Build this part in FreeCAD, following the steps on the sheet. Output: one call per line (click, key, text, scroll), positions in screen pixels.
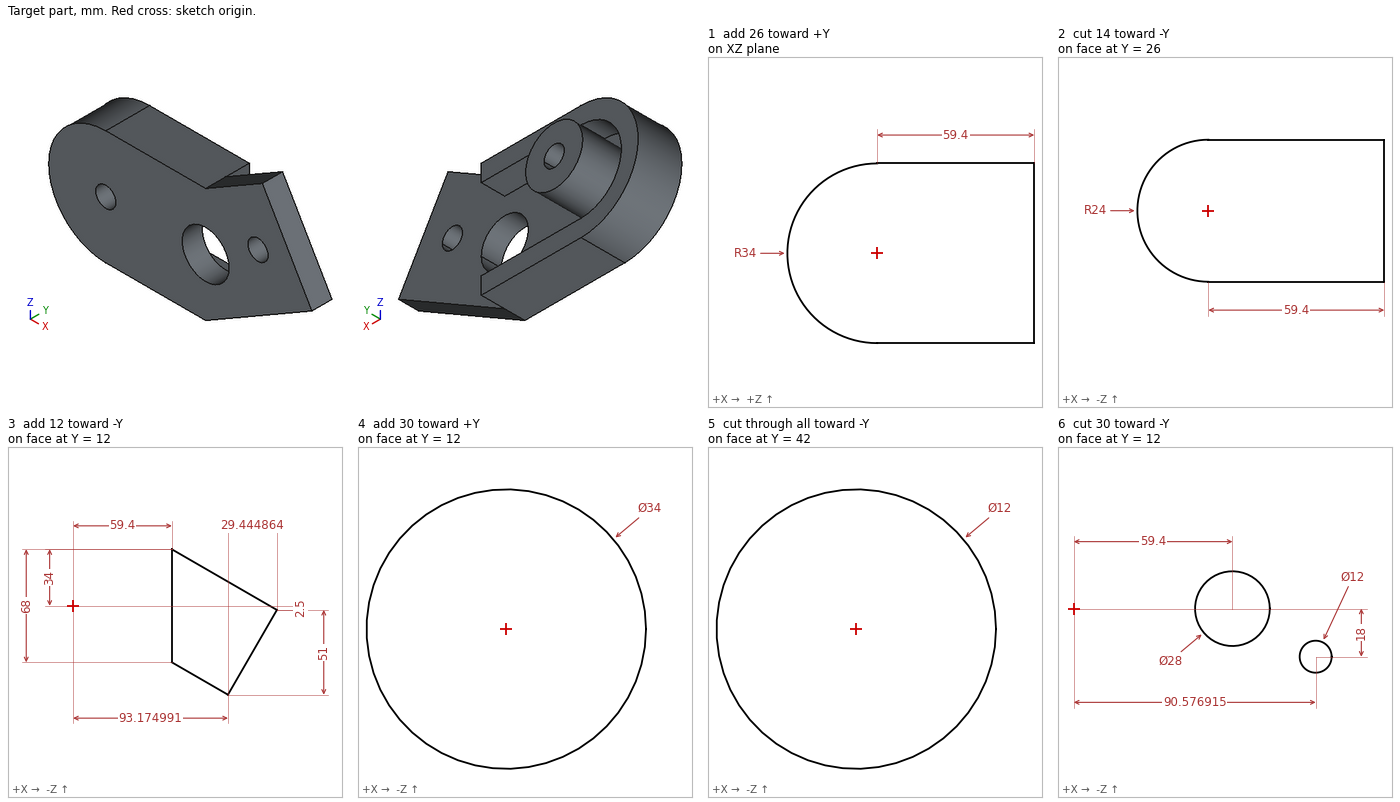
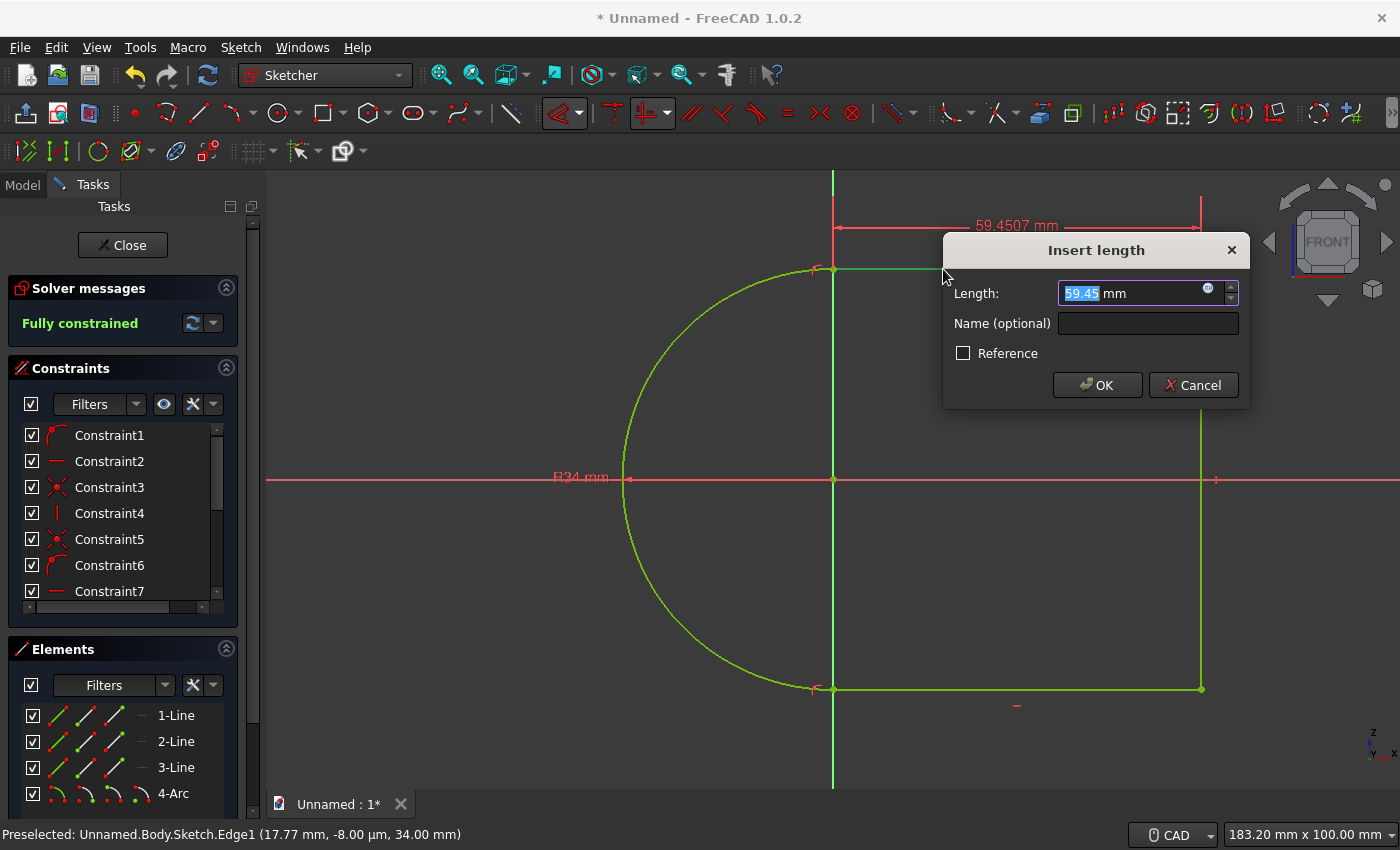
text(59.4)
key(Return)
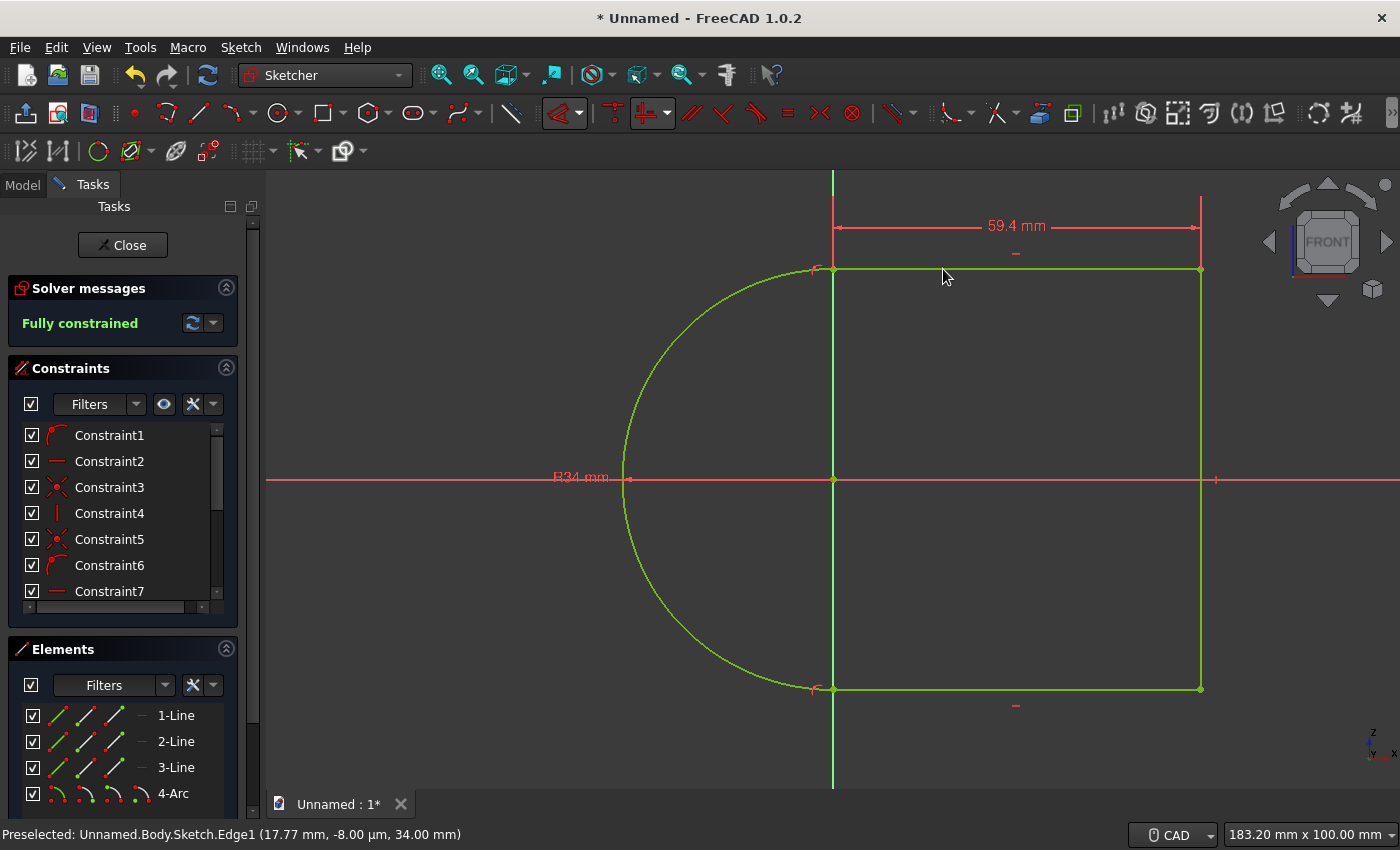
click(123, 245)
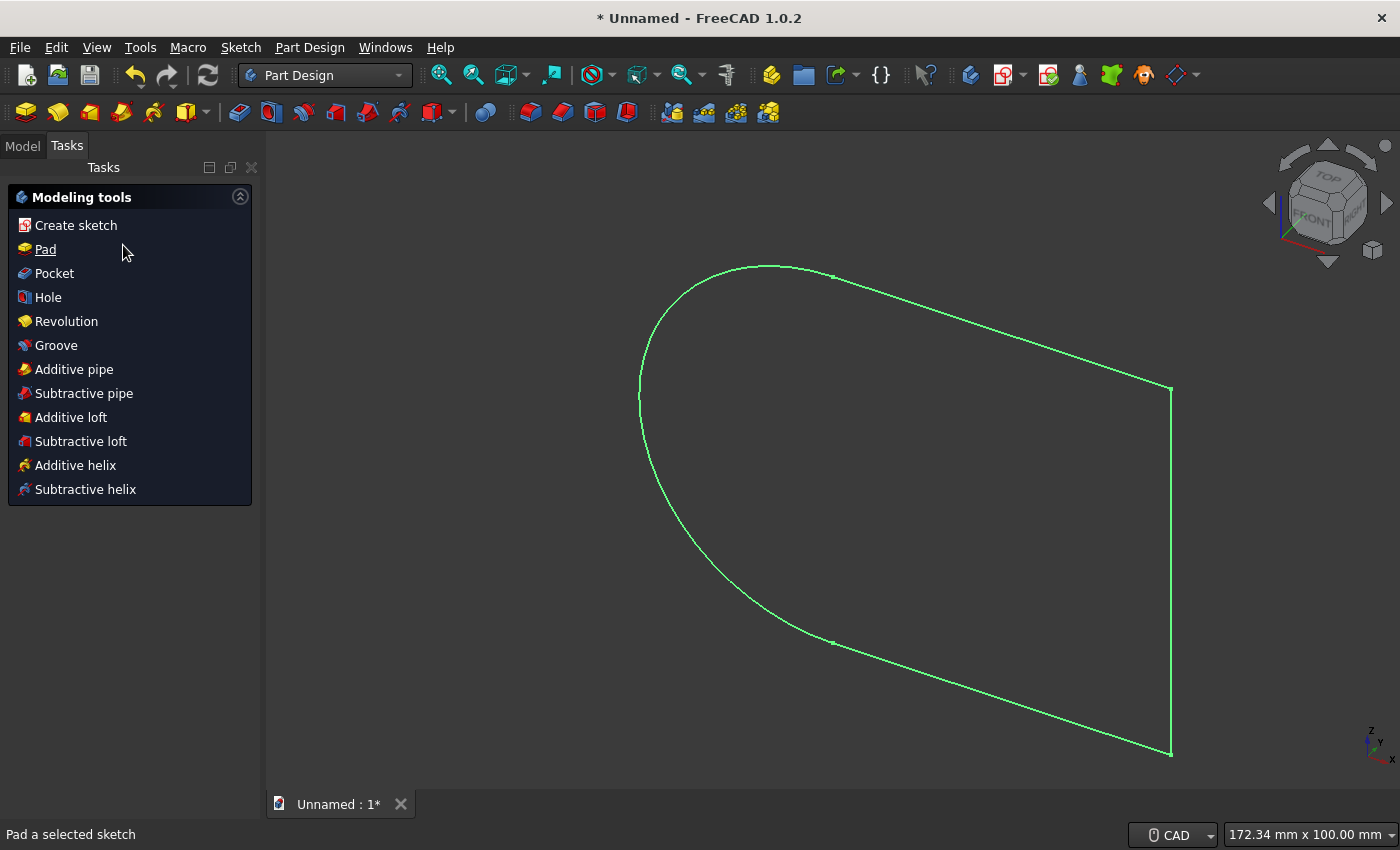
click(26, 112)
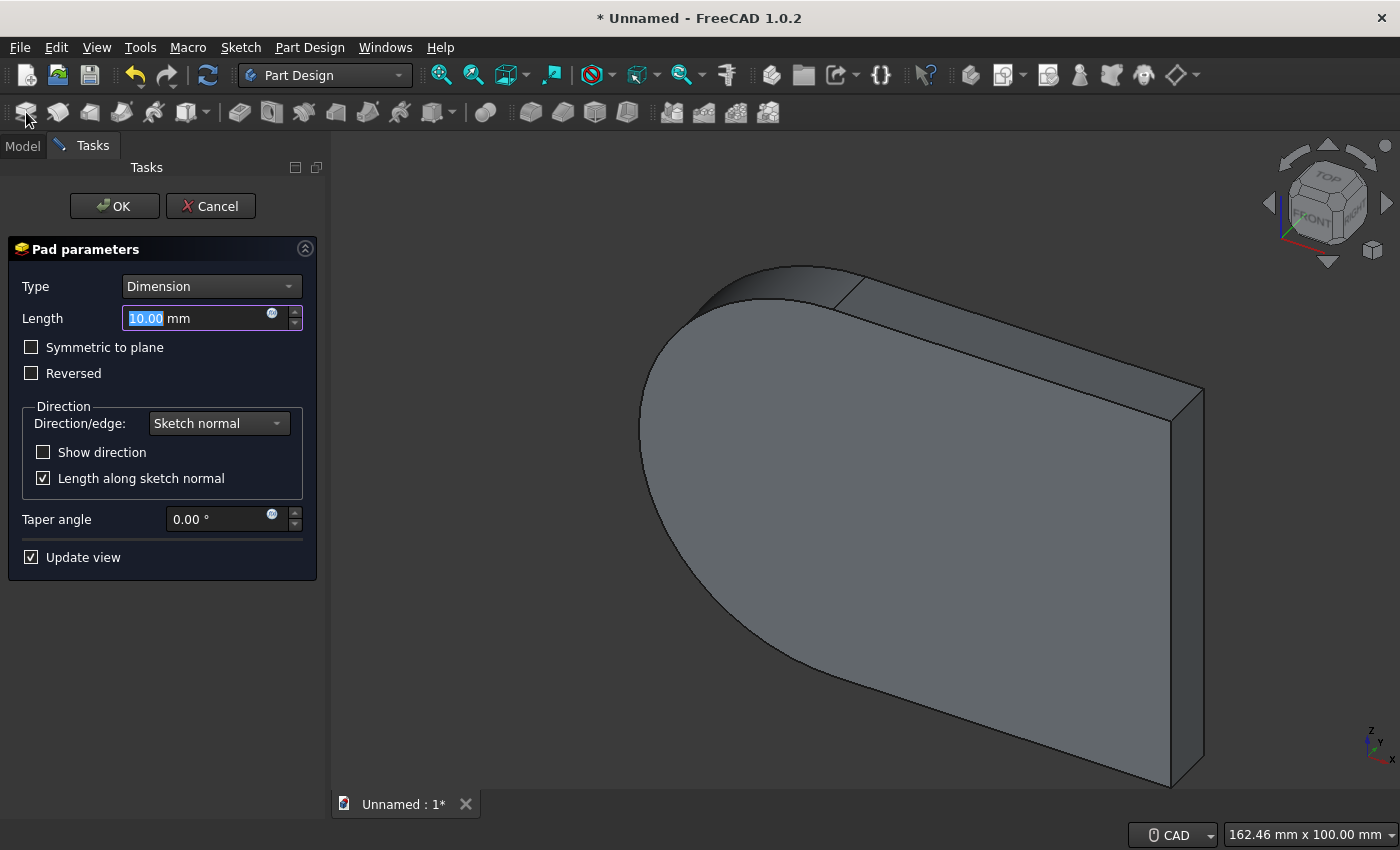
text(26)
key(Tab)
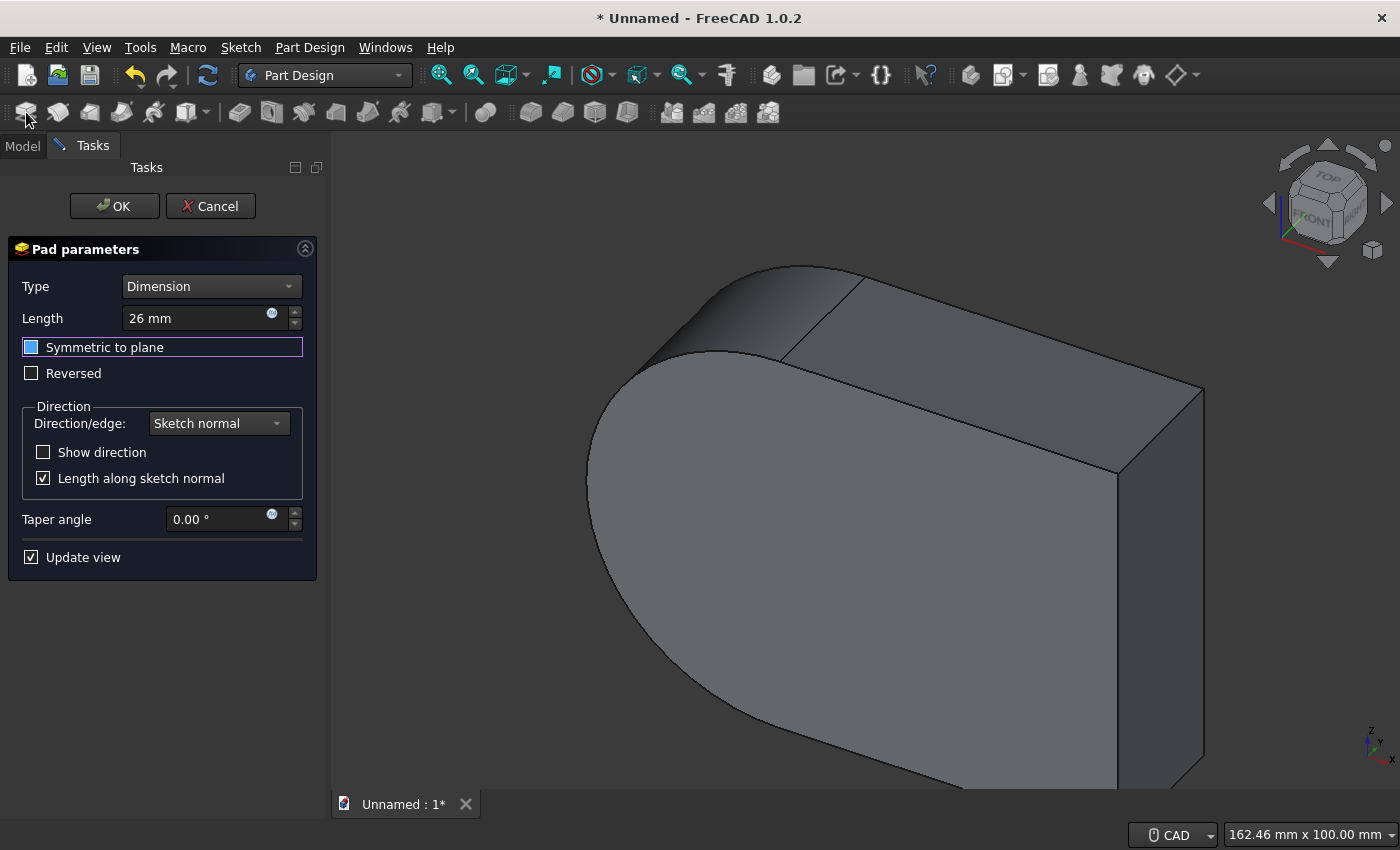
click(30, 373)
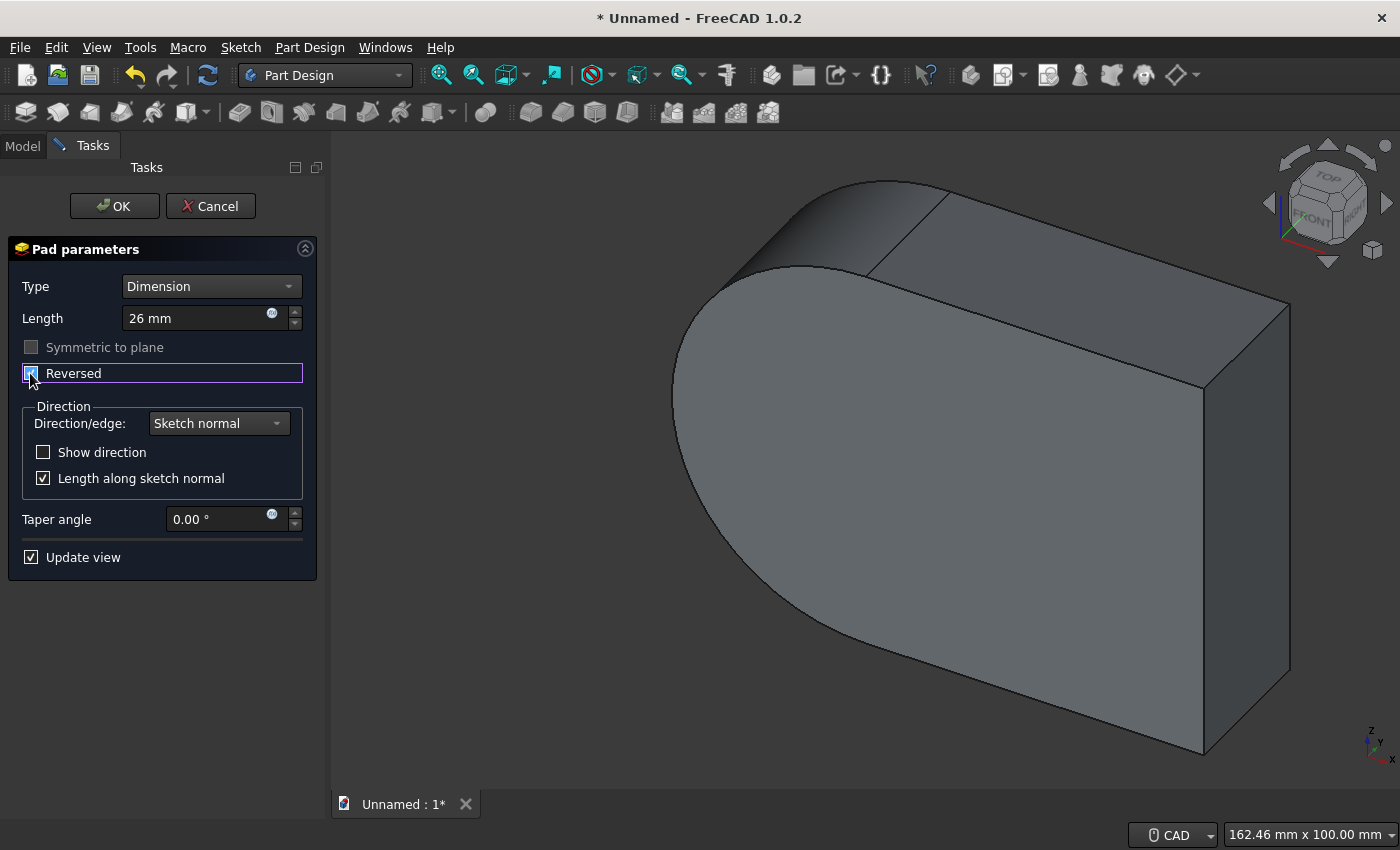
click(115, 206)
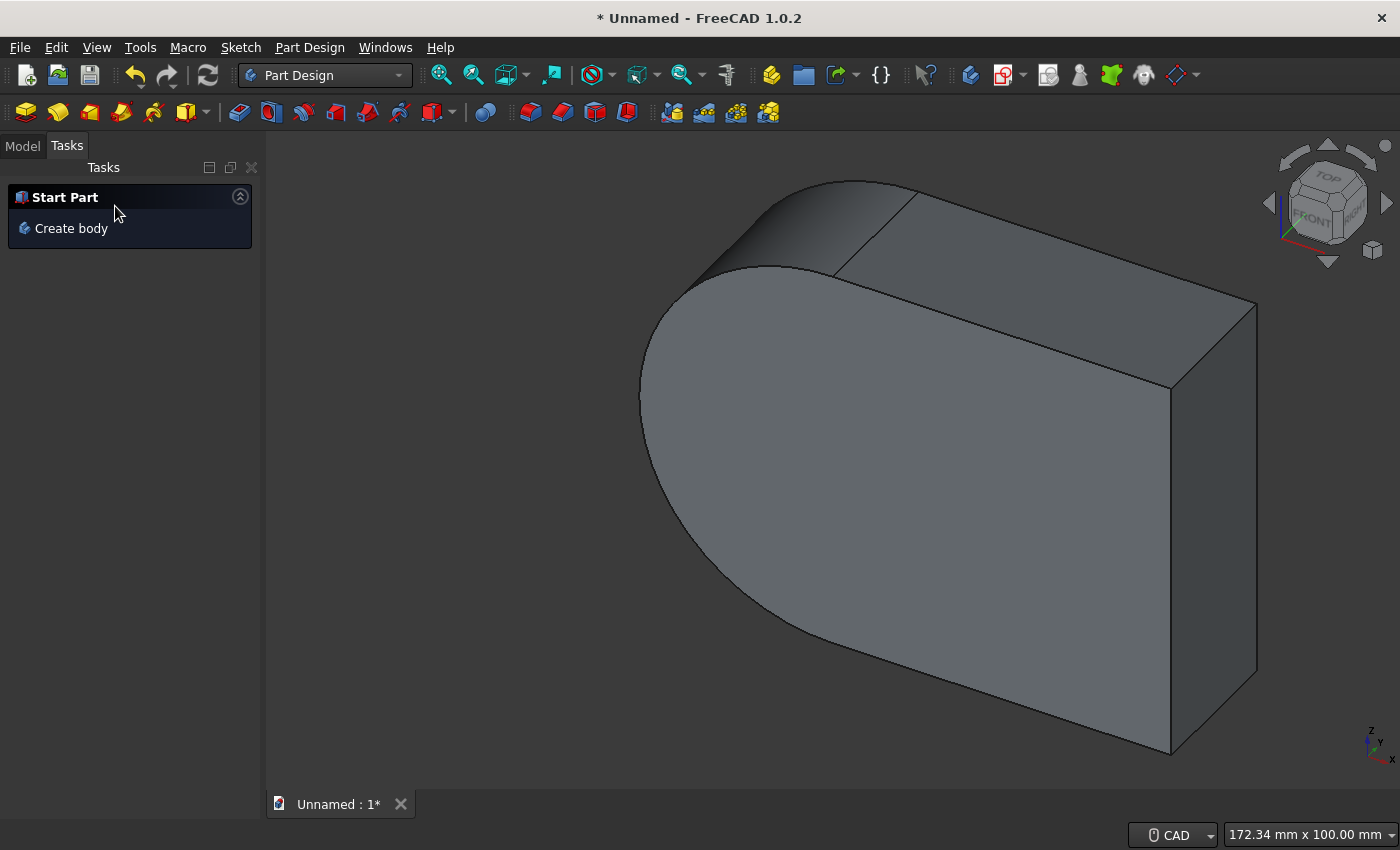
click(442, 76)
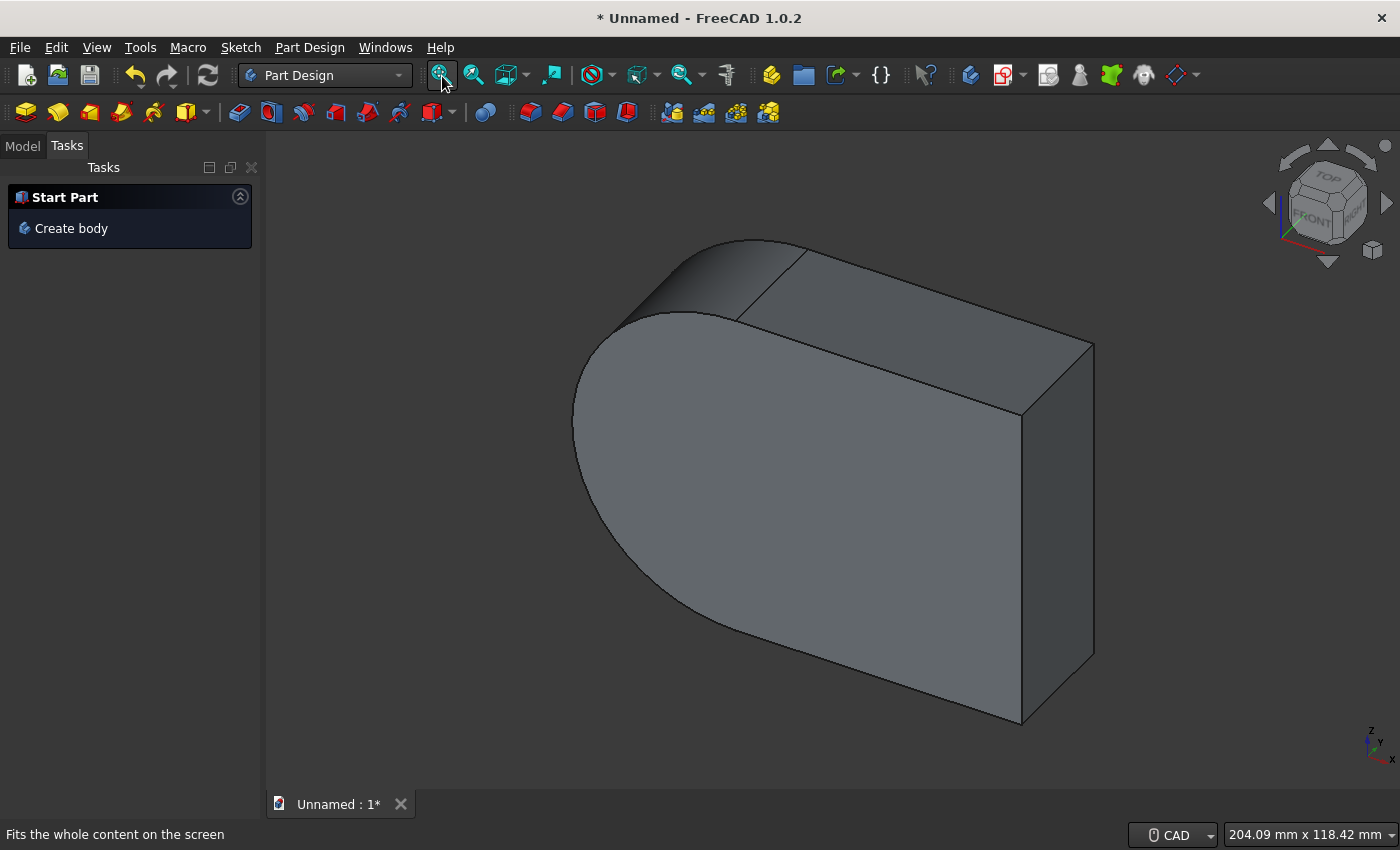
key(4)